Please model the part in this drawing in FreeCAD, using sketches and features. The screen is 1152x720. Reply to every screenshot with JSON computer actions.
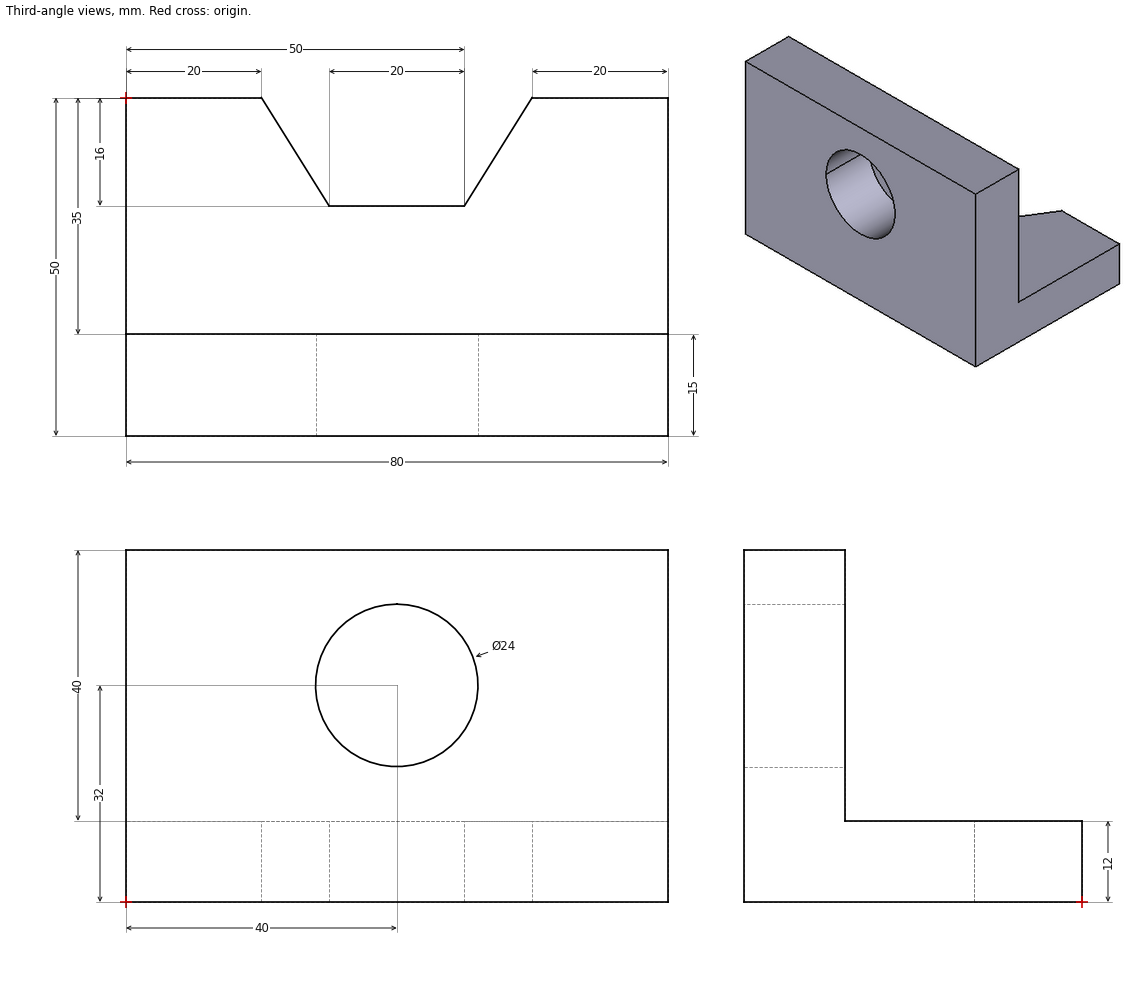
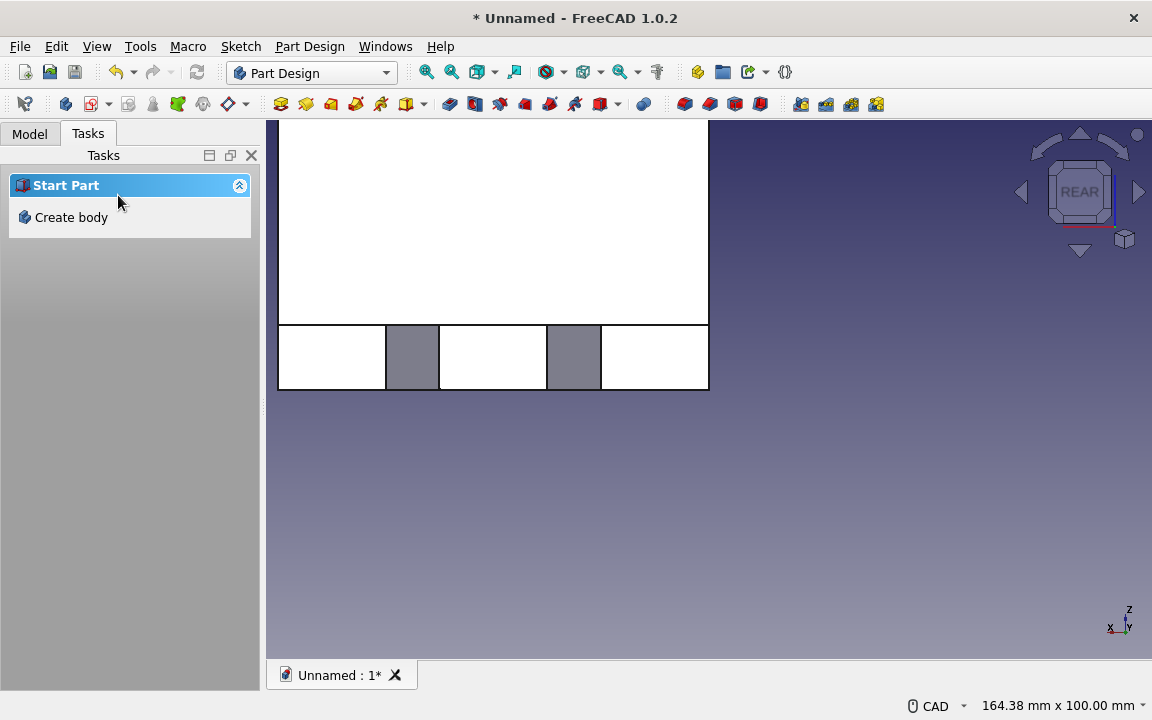
{"action": "key", "text": "v f"}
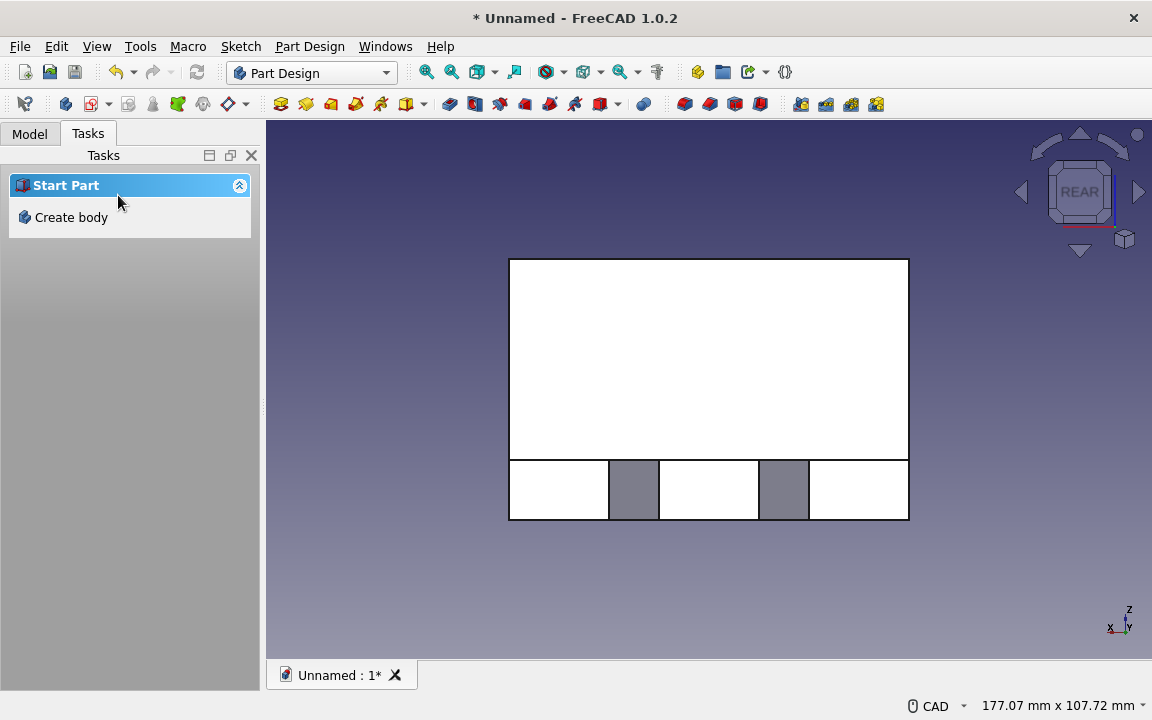
{"action": "left_click", "coordinate": [652, 358]}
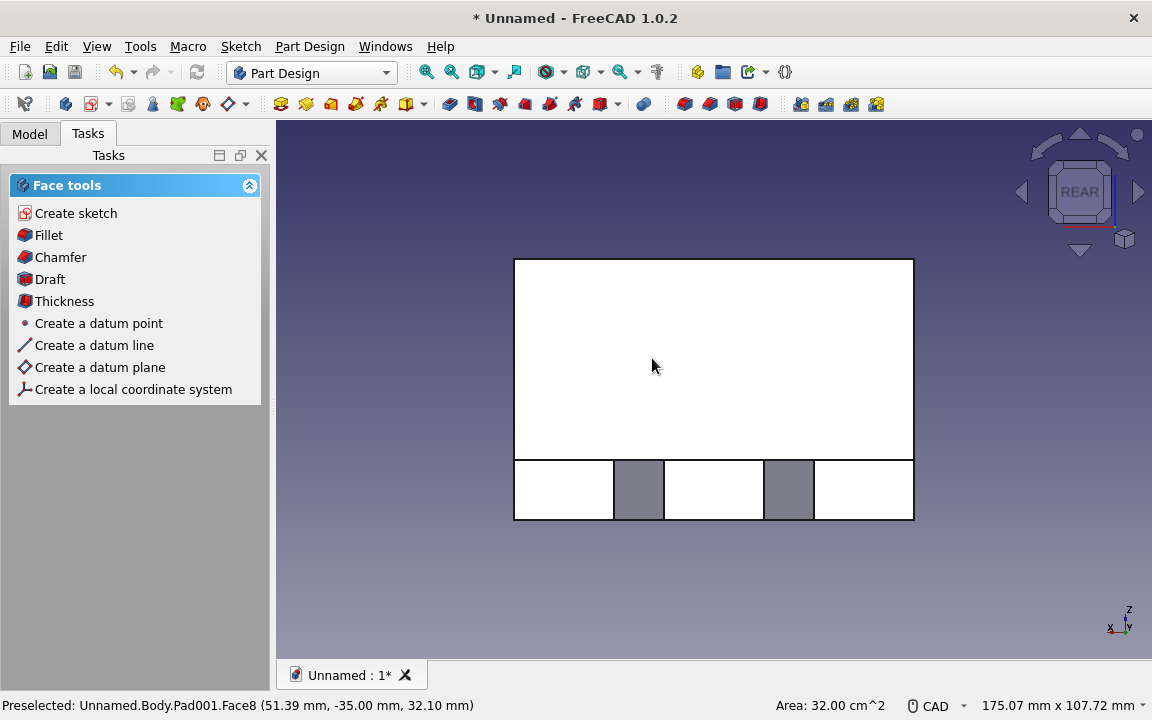
{"action": "left_click", "coordinate": [90, 104]}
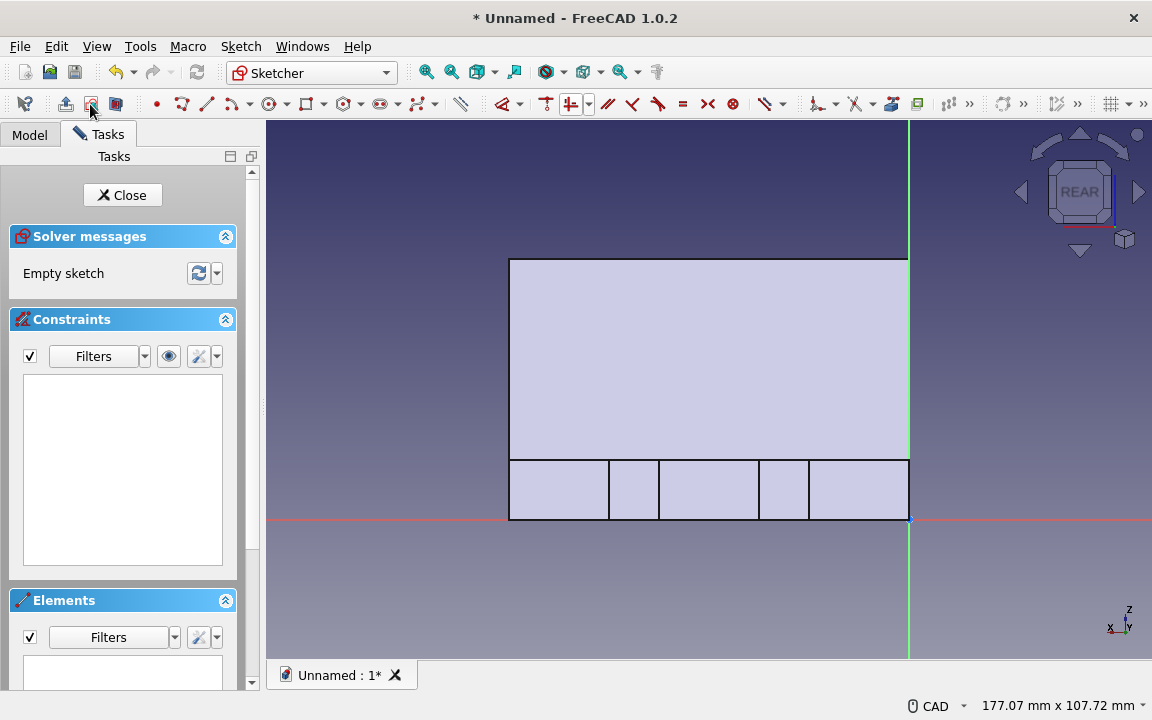
{"action": "left_click", "coordinate": [116, 104]}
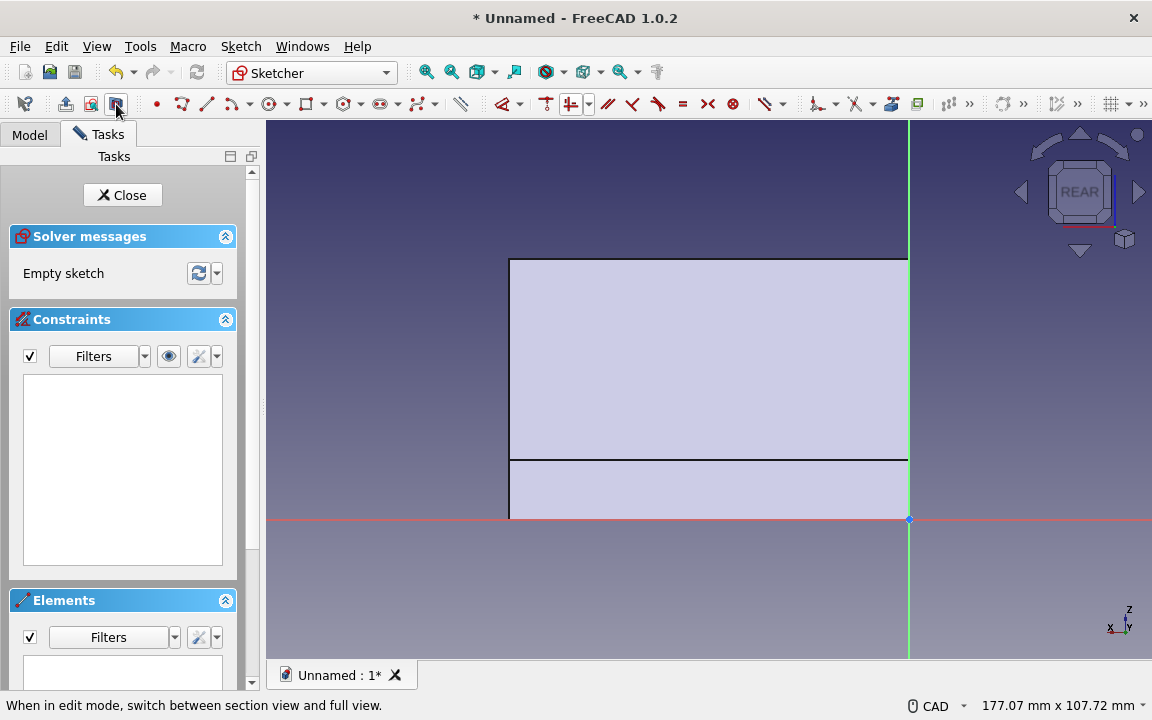
{"action": "scroll", "coordinate": [987, 450], "scroll_direction": "up", "scroll_amount": 2}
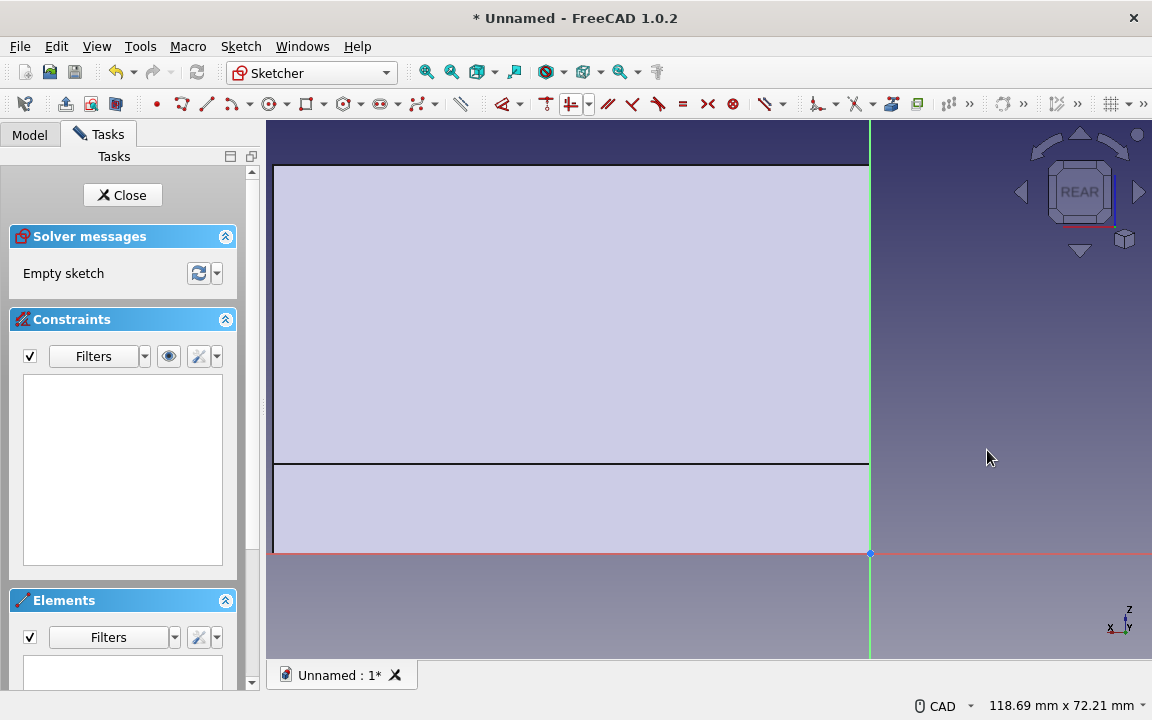
{"action": "left_click", "coordinate": [268, 104]}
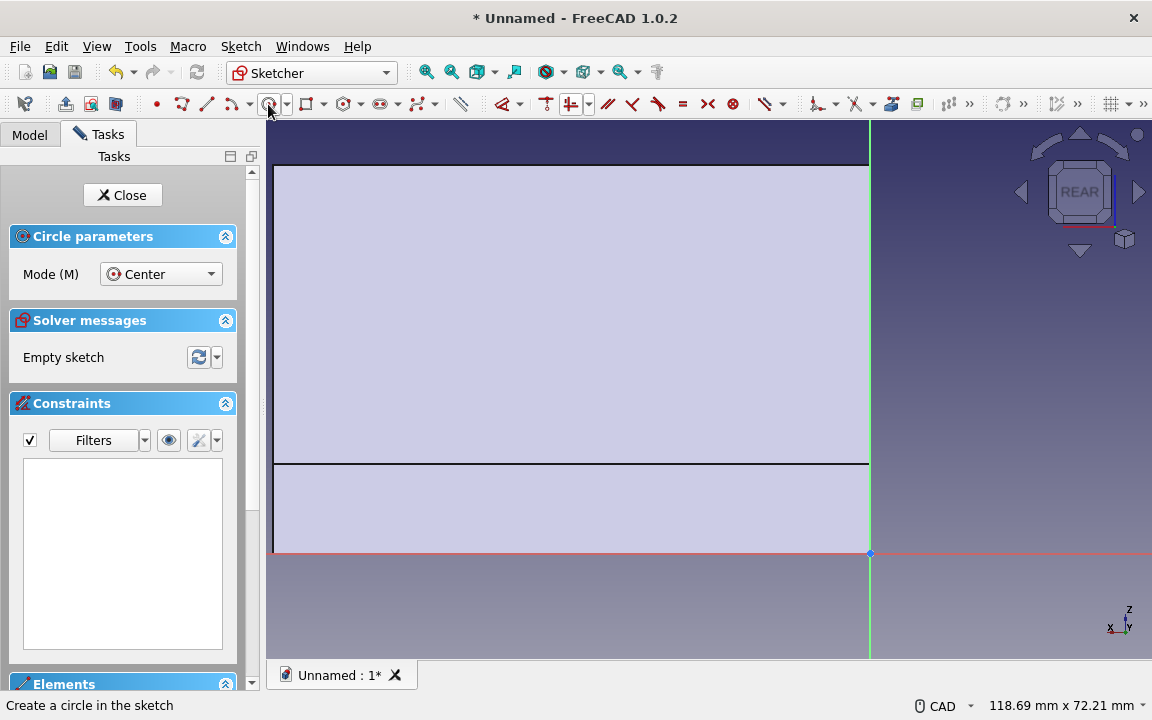
{"action": "left_click", "coordinate": [572, 315]}
{"action": "mouse_move", "coordinate": [635, 251]}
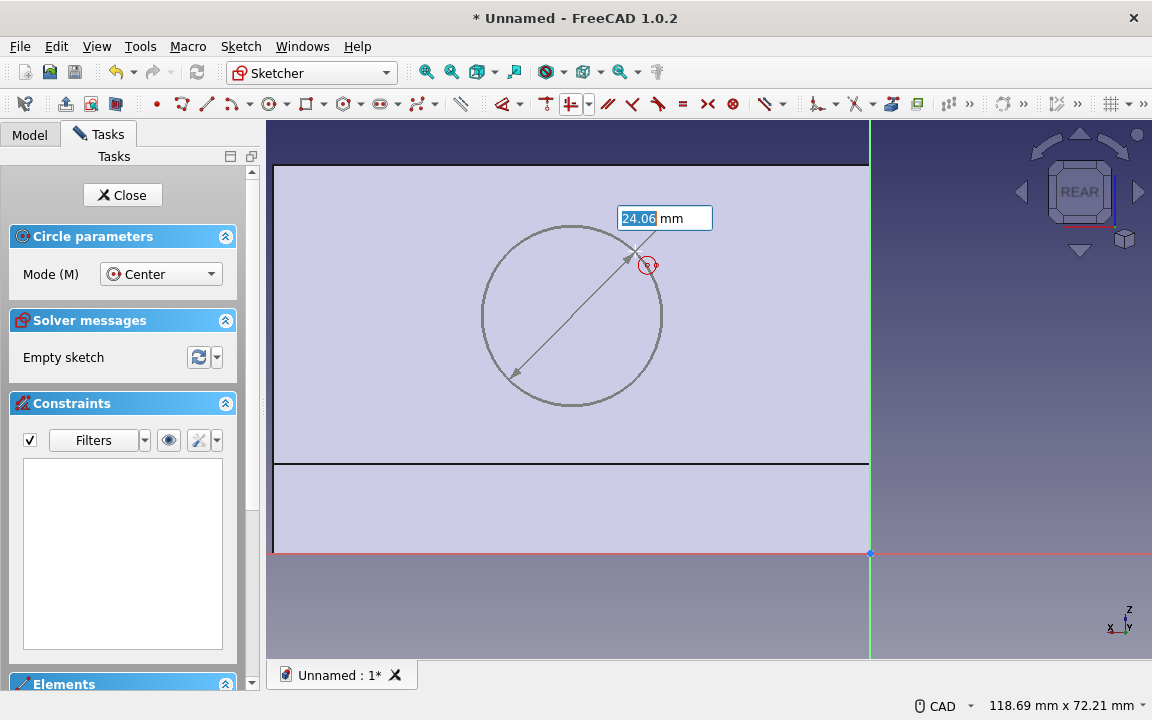
{"action": "type", "text": "24"}
{"action": "key", "text": "Return"}
{"action": "key", "text": "Escape"}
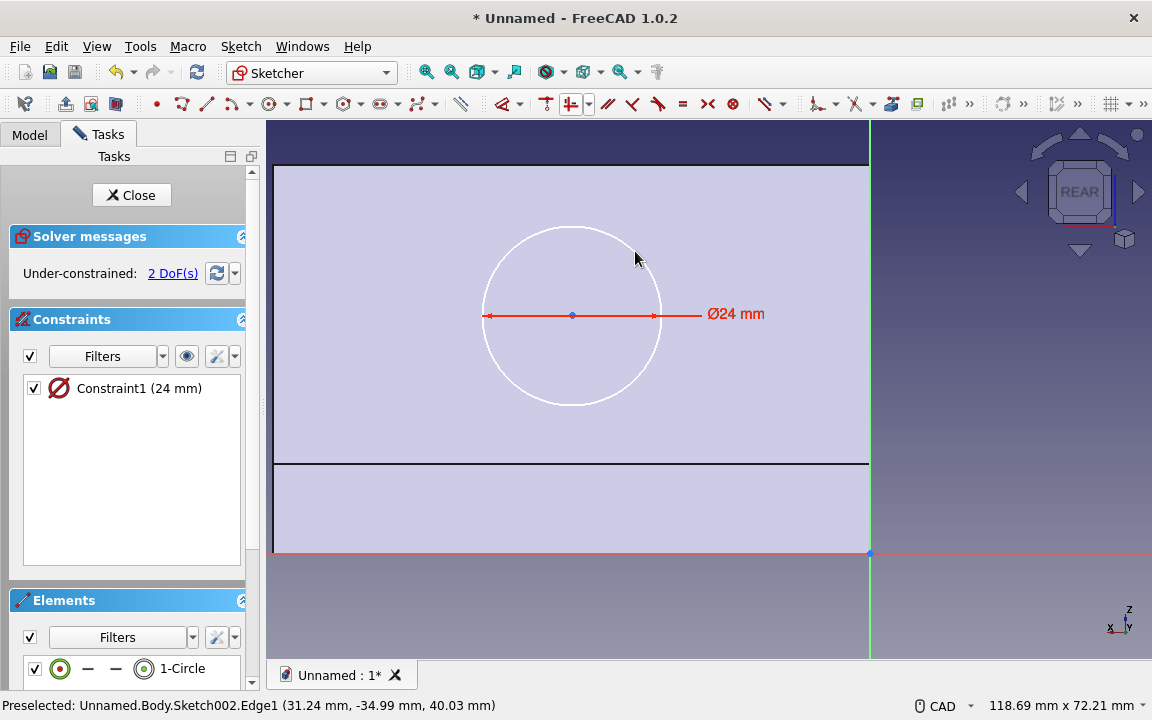
{"action": "left_click", "coordinate": [502, 104]}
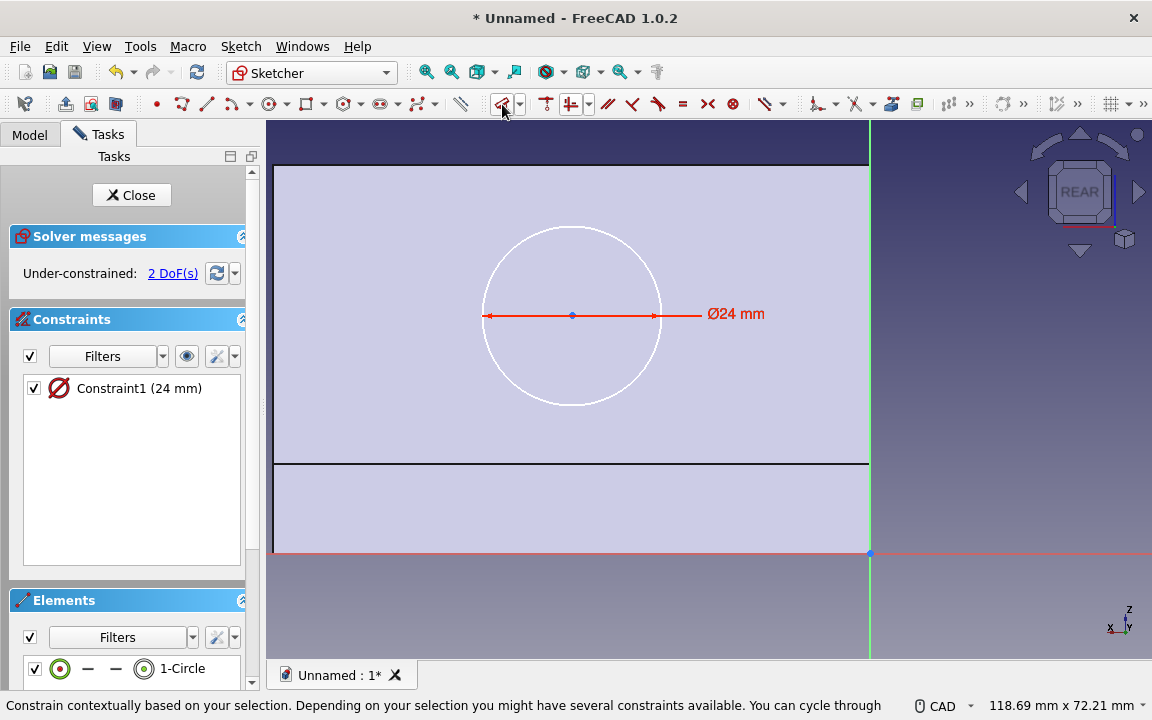
{"action": "left_click", "coordinate": [572, 316]}
{"action": "left_click", "coordinate": [721, 588]}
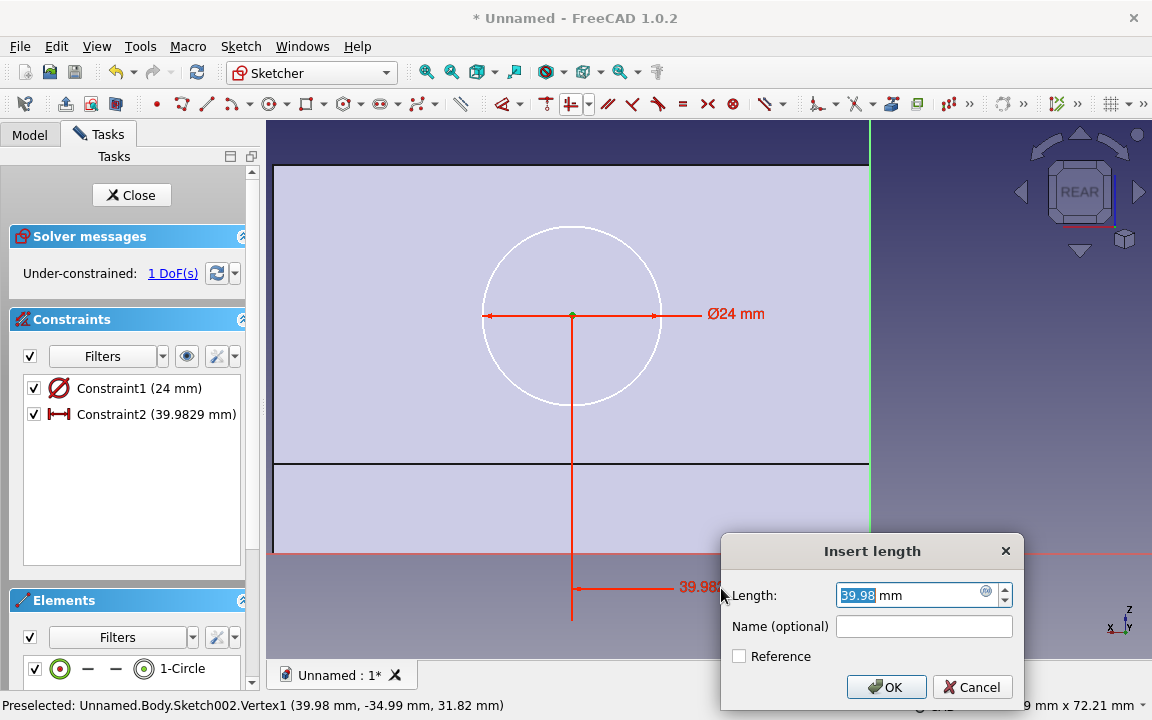
{"action": "type", "text": "40"}
{"action": "key", "text": "Return"}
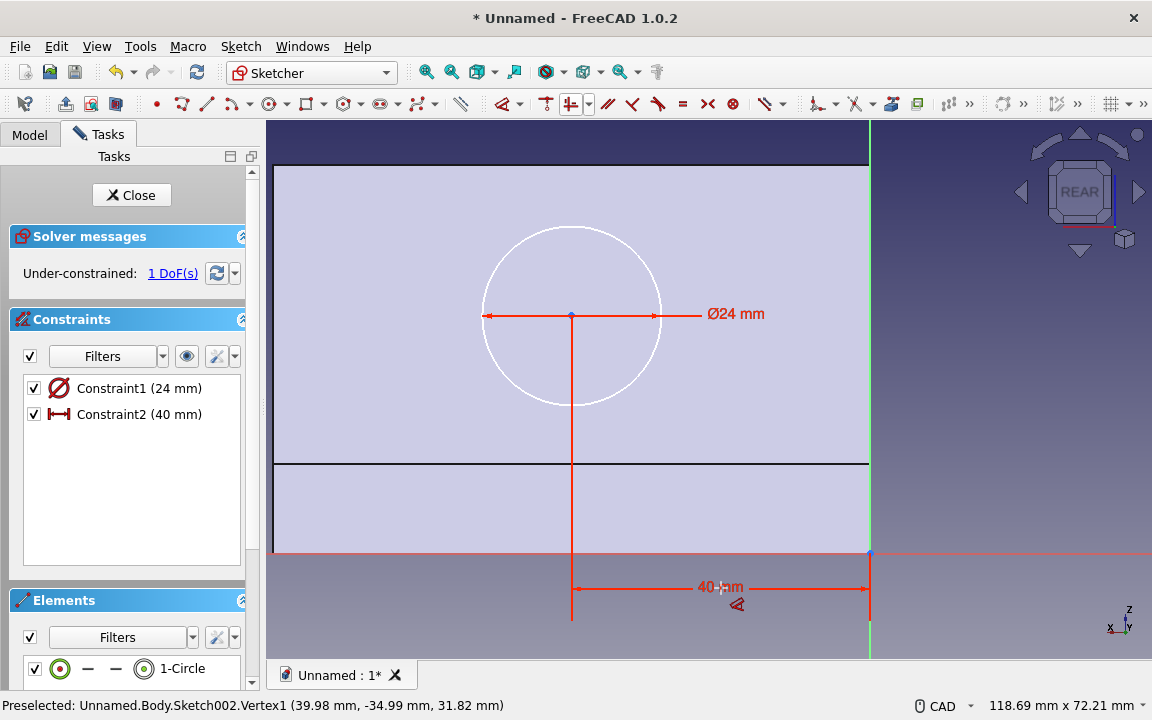
{"action": "left_click", "coordinate": [572, 316]}
{"action": "left_click", "coordinate": [904, 435]}